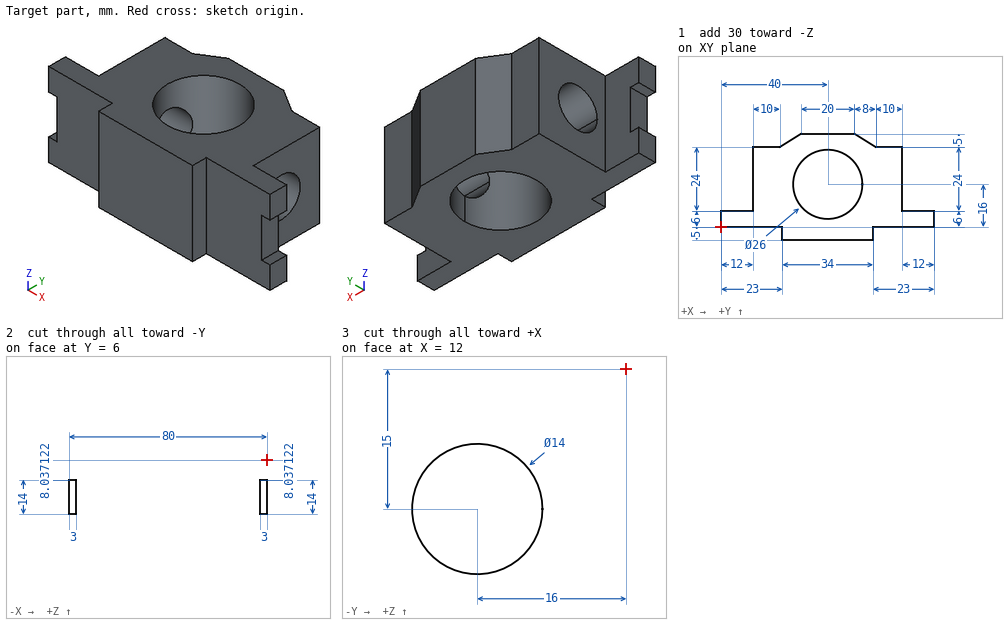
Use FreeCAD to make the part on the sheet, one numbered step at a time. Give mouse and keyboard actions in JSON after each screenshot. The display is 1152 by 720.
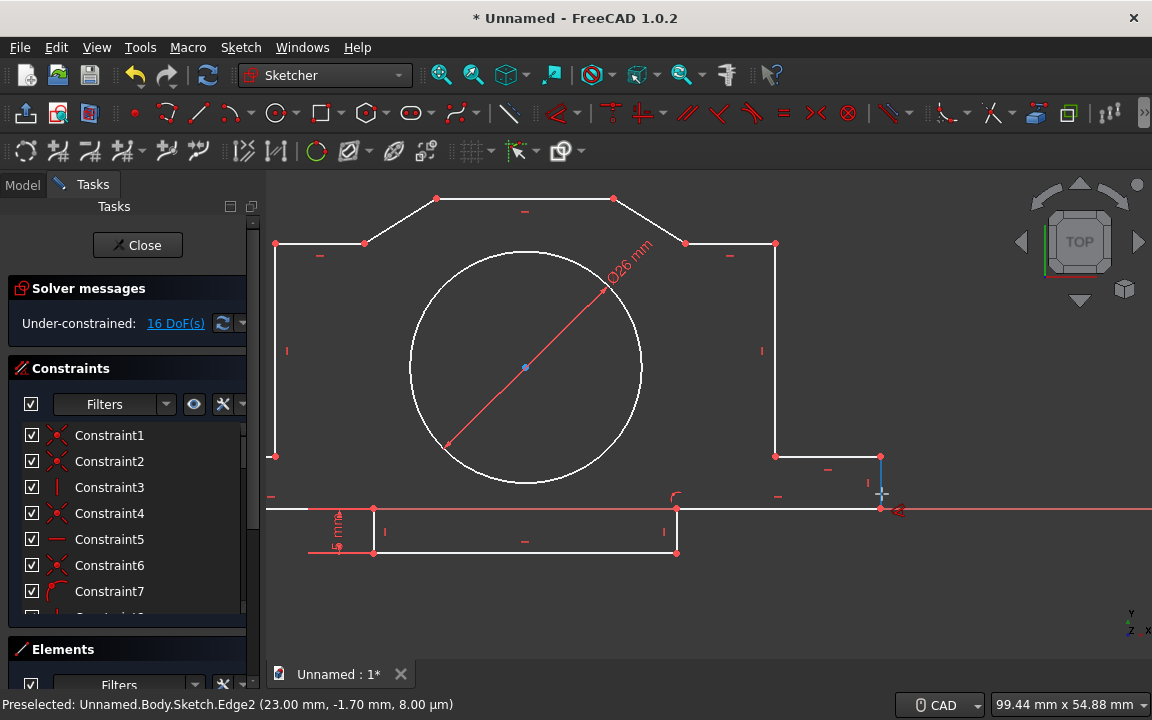
{"action": "left_click", "coordinate": [881, 493]}
{"action": "left_click", "coordinate": [915, 483]}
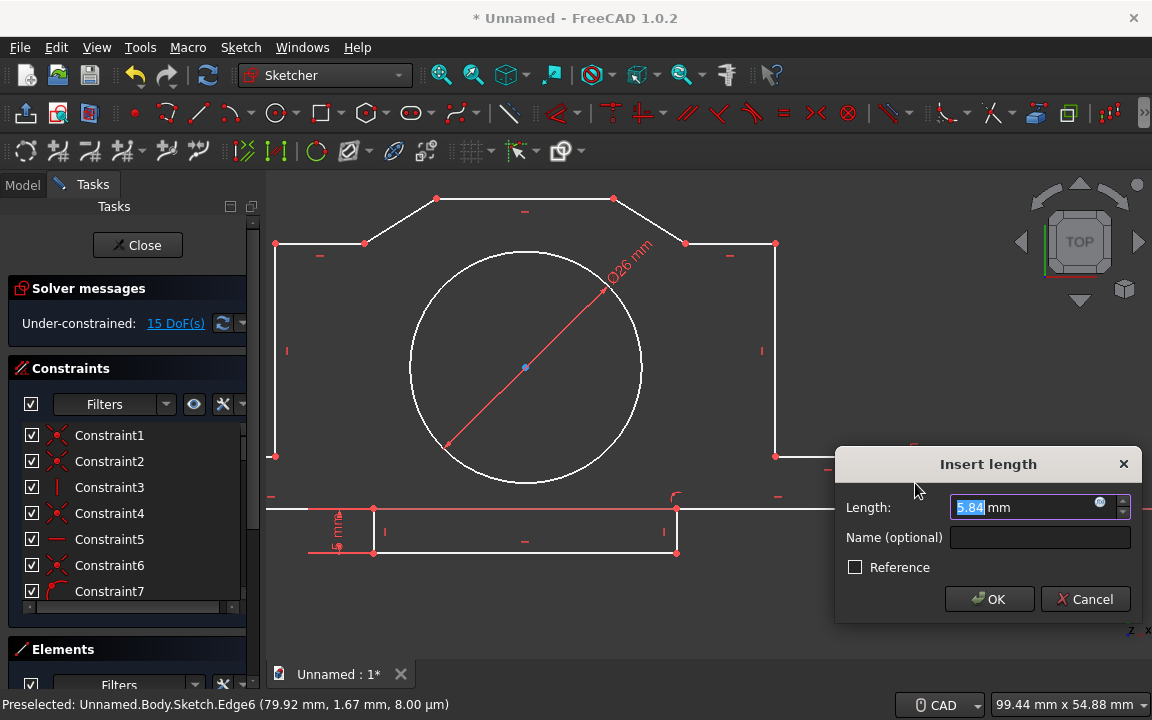
{"action": "type", "text": "6"}
{"action": "key", "text": "Return"}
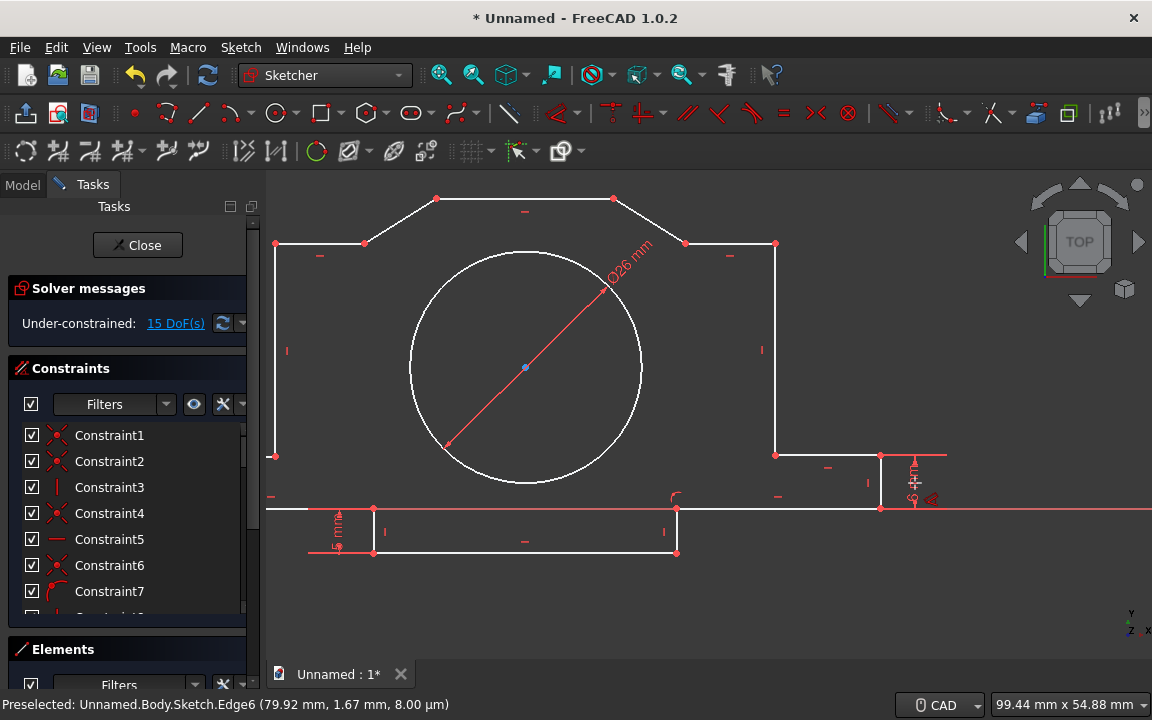
{"action": "scroll", "coordinate": [875, 494], "scroll_direction": "down", "scroll_amount": 2}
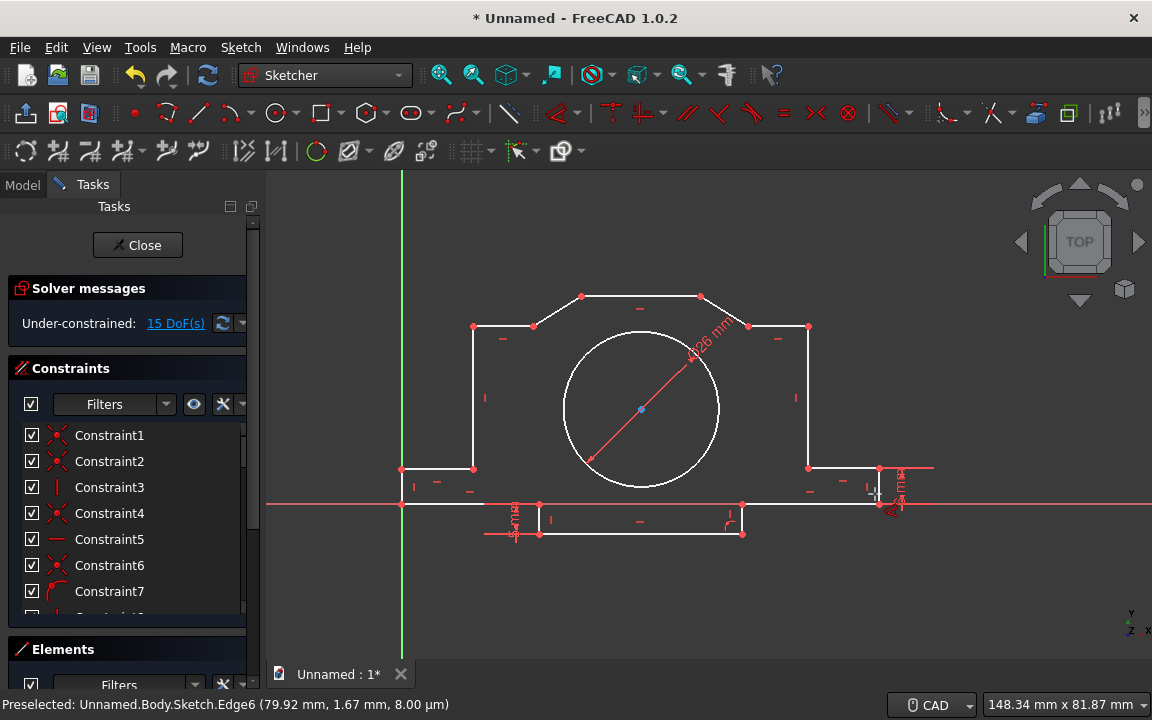
{"action": "scroll", "coordinate": [402, 480], "scroll_direction": "up", "scroll_amount": 2}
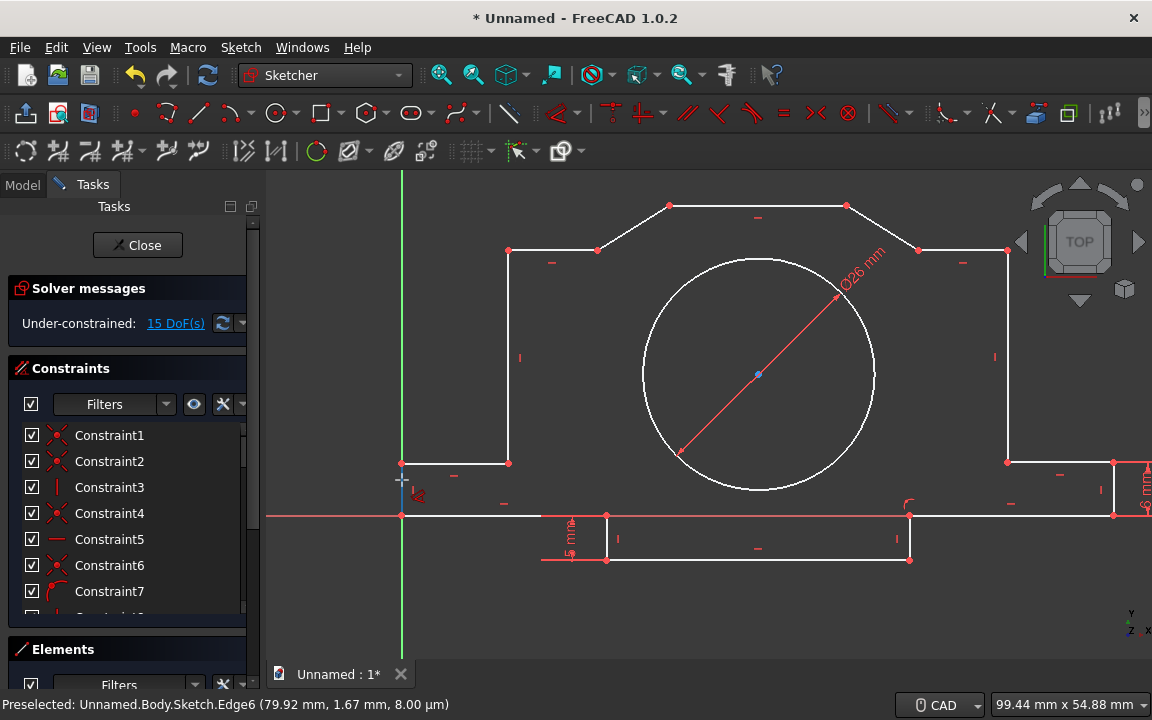
{"action": "left_click", "coordinate": [402, 479]}
{"action": "left_click", "coordinate": [368, 490]}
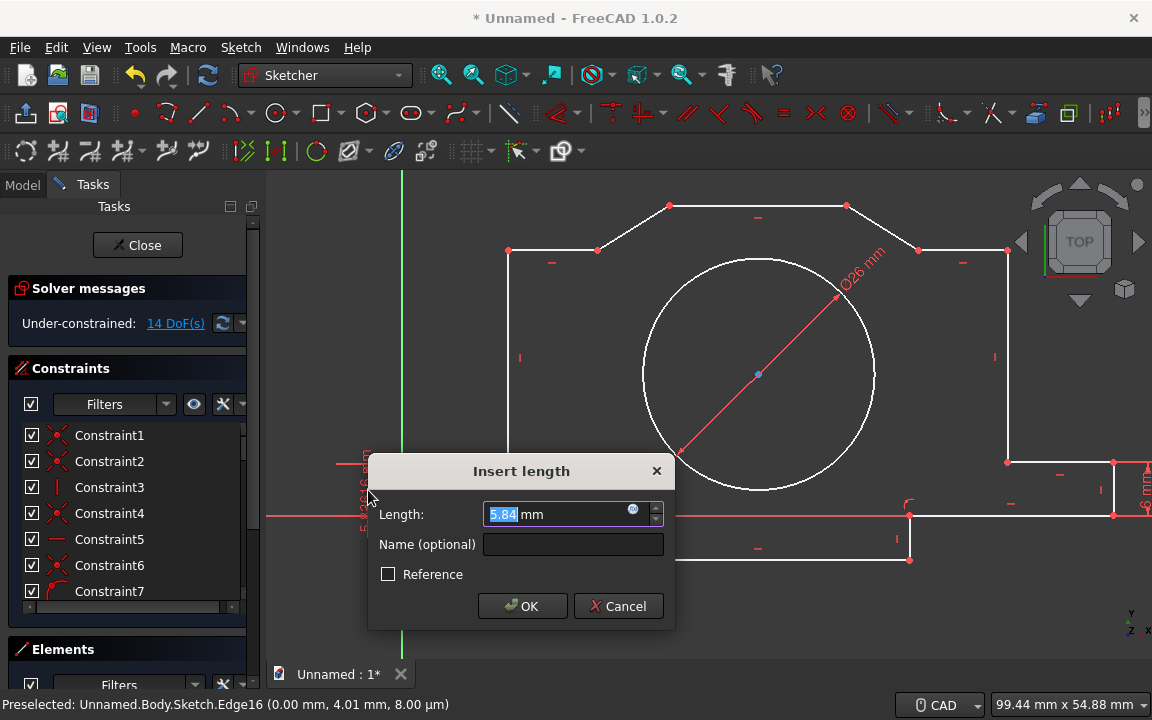
{"action": "type", "text": "6"}
{"action": "key", "text": "Return"}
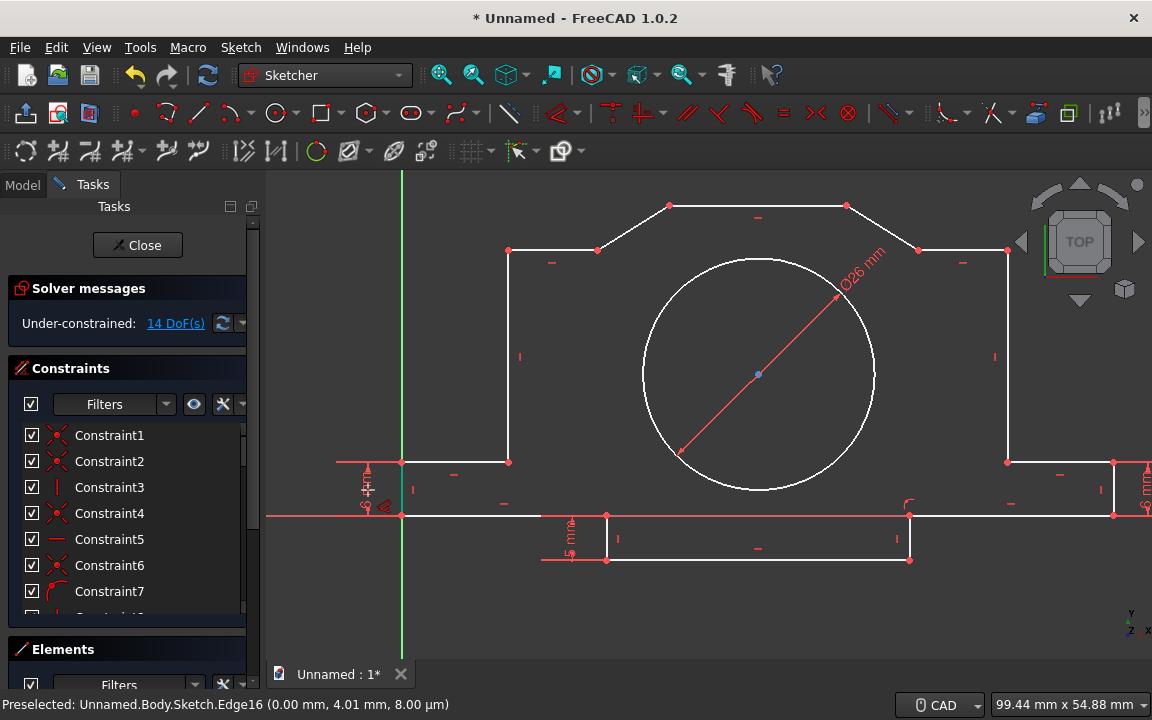
{"action": "left_click", "coordinate": [463, 516]}
{"action": "left_click", "coordinate": [457, 550]}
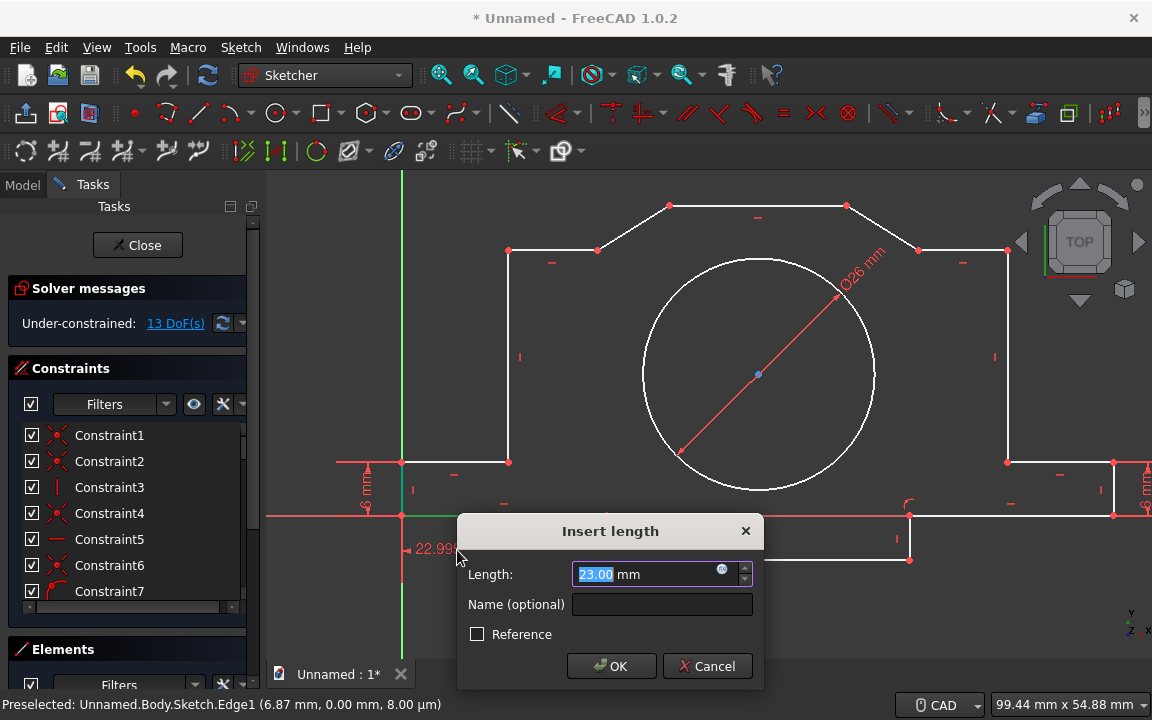
{"action": "type", "text": "23"}
{"action": "key", "text": "Return"}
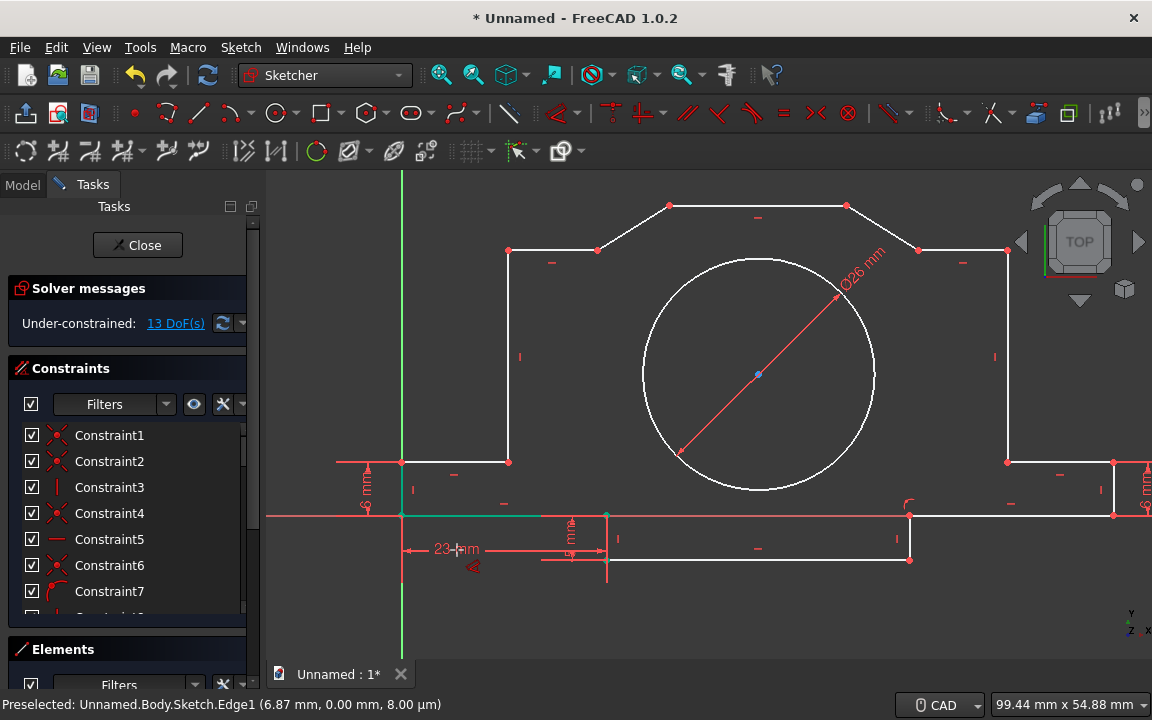
{"action": "left_click", "coordinate": [698, 560]}
{"action": "left_click", "coordinate": [758, 594]}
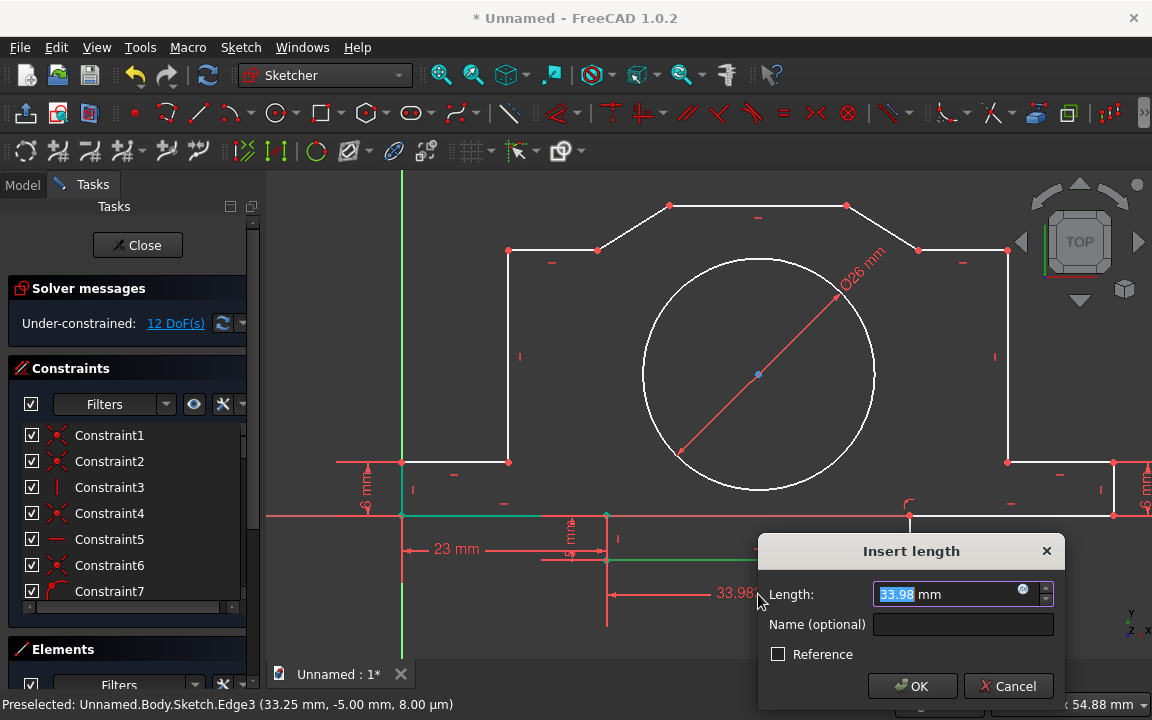
{"action": "type", "text": "34"}
{"action": "key", "text": "Return"}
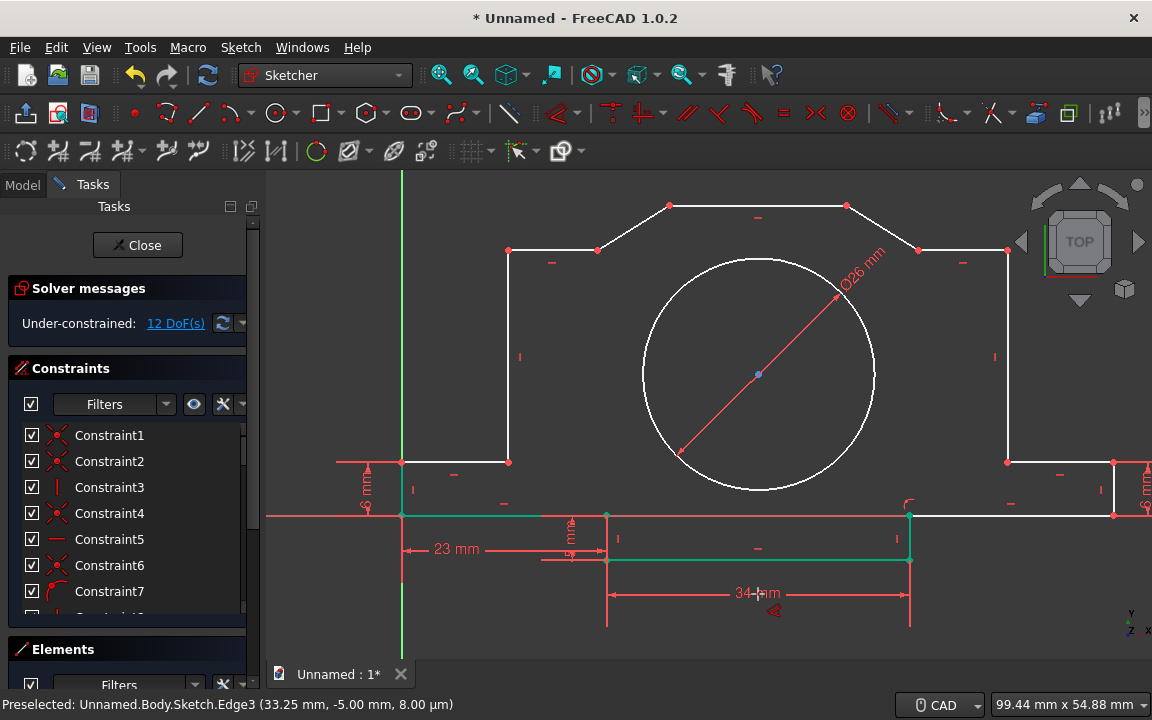
{"action": "left_click", "coordinate": [971, 516]}
{"action": "left_click", "coordinate": [948, 550]}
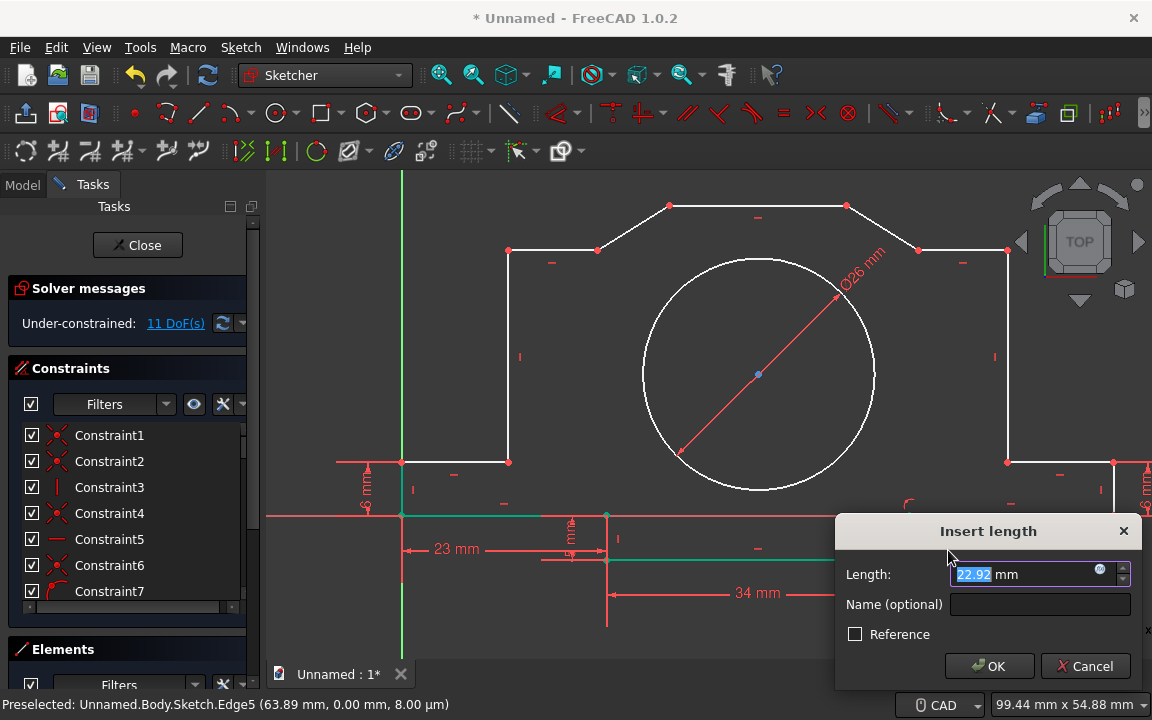
{"action": "type", "text": "23"}
{"action": "key", "text": "Return"}